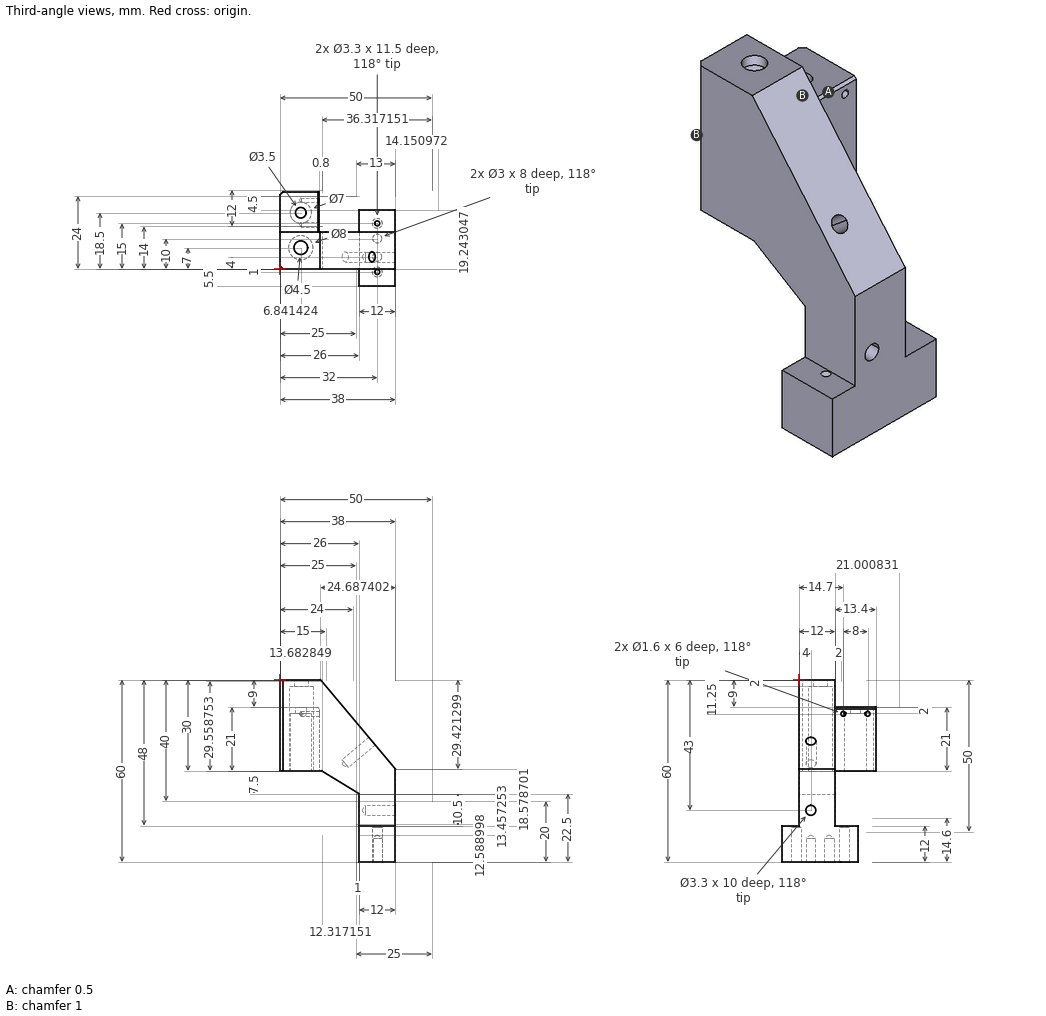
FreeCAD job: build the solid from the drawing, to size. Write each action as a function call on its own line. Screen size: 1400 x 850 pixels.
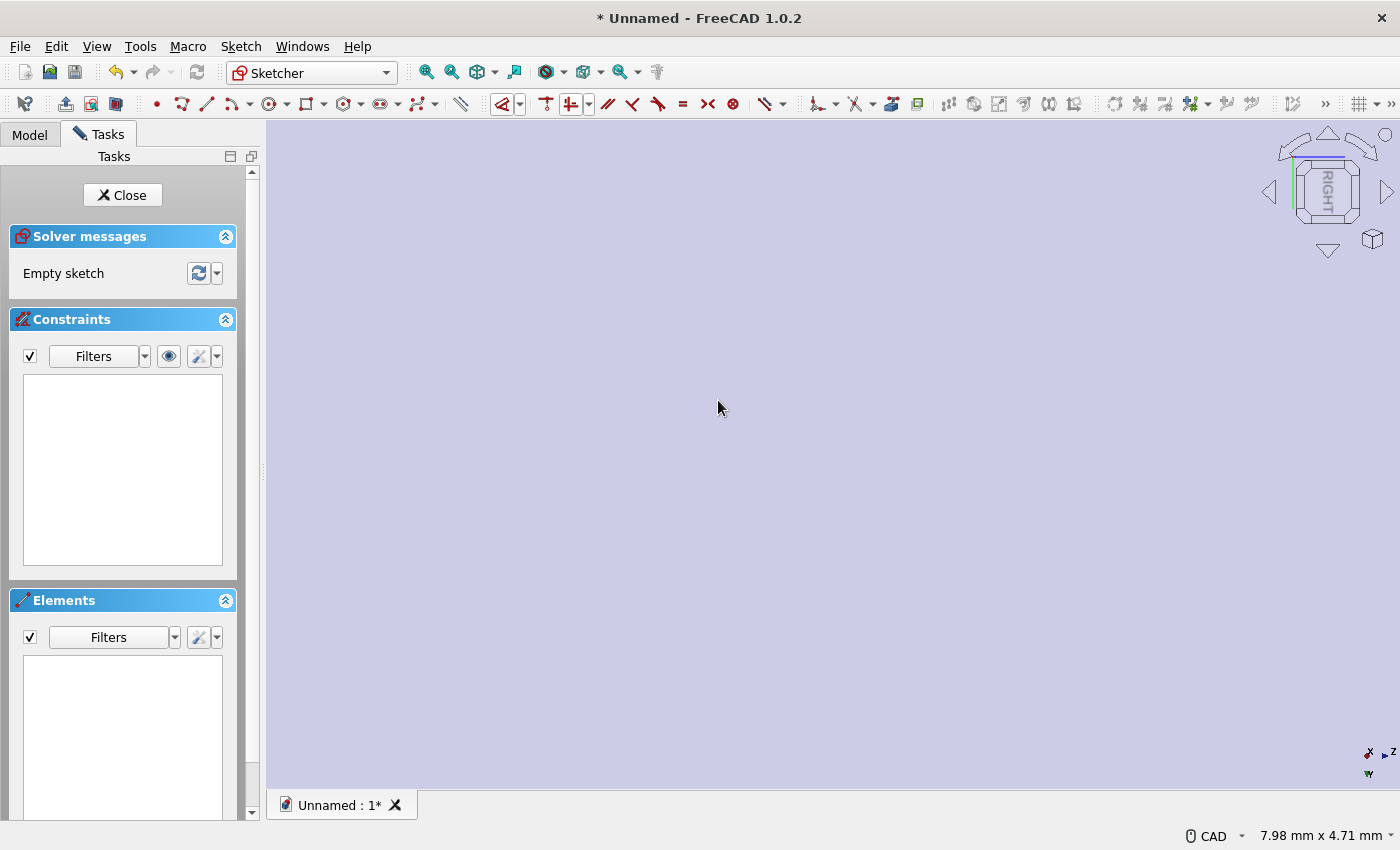
click(268, 104)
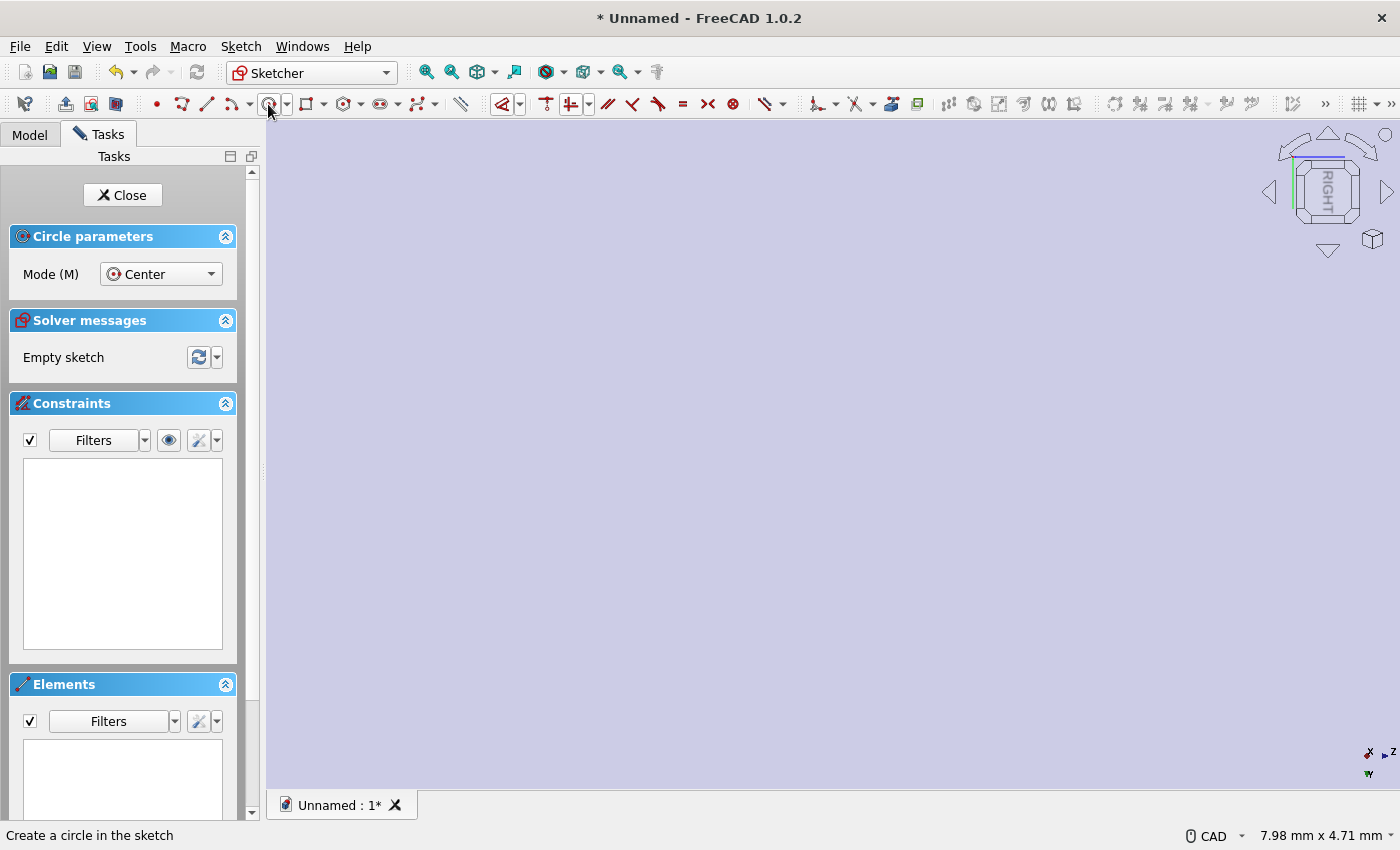
click(756, 445)
click(922, 279)
key(Escape)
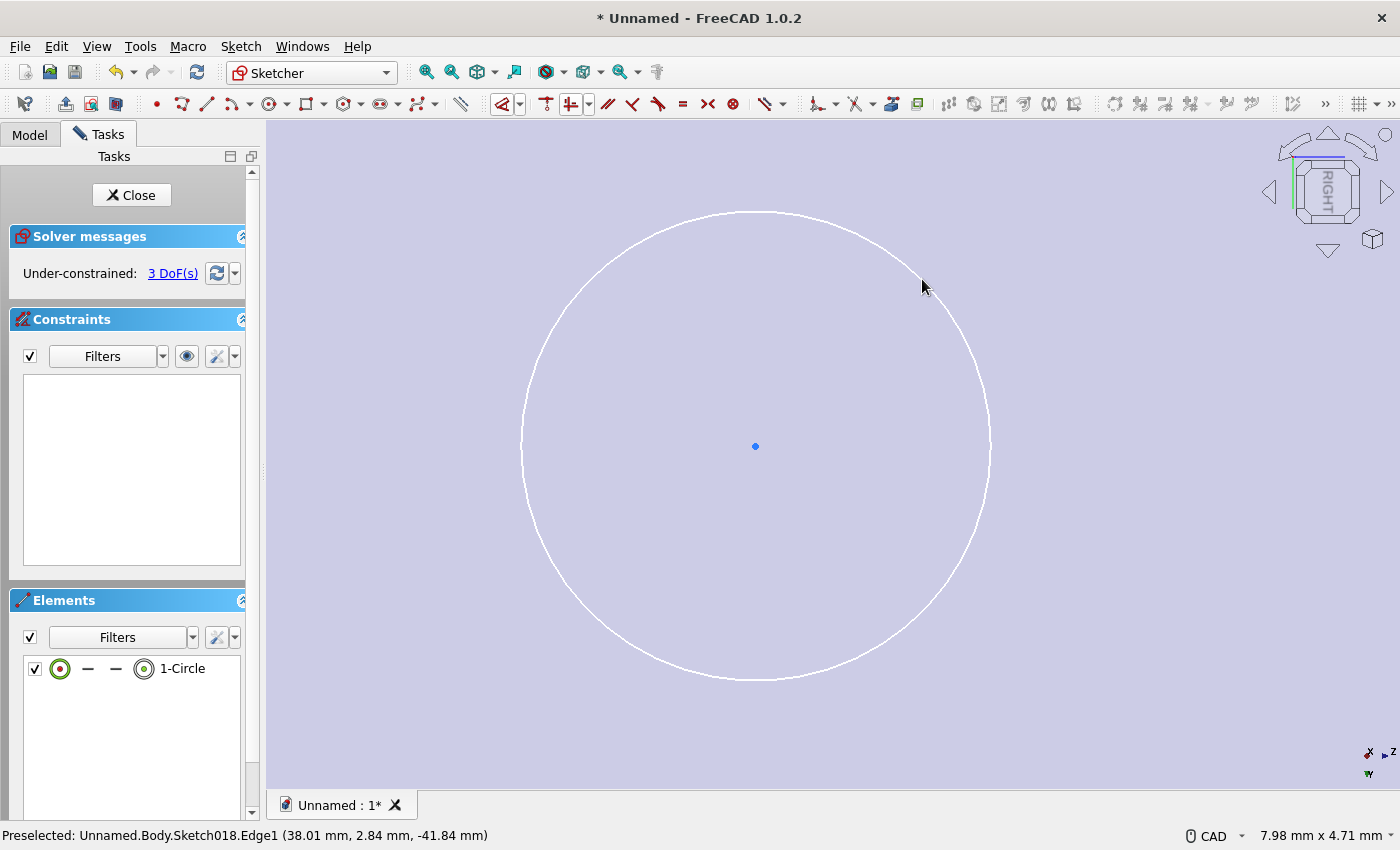
click(921, 279)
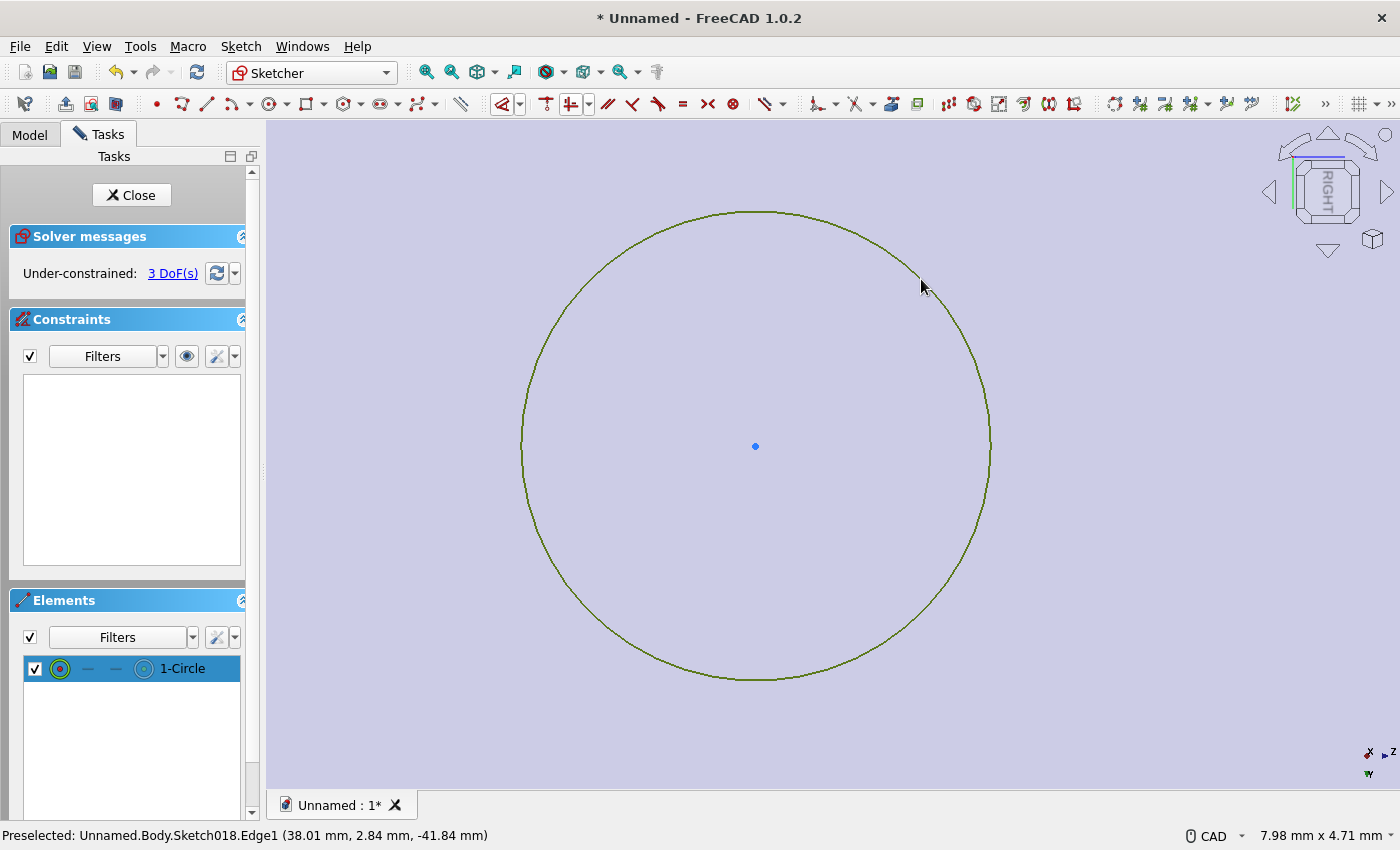
click(520, 104)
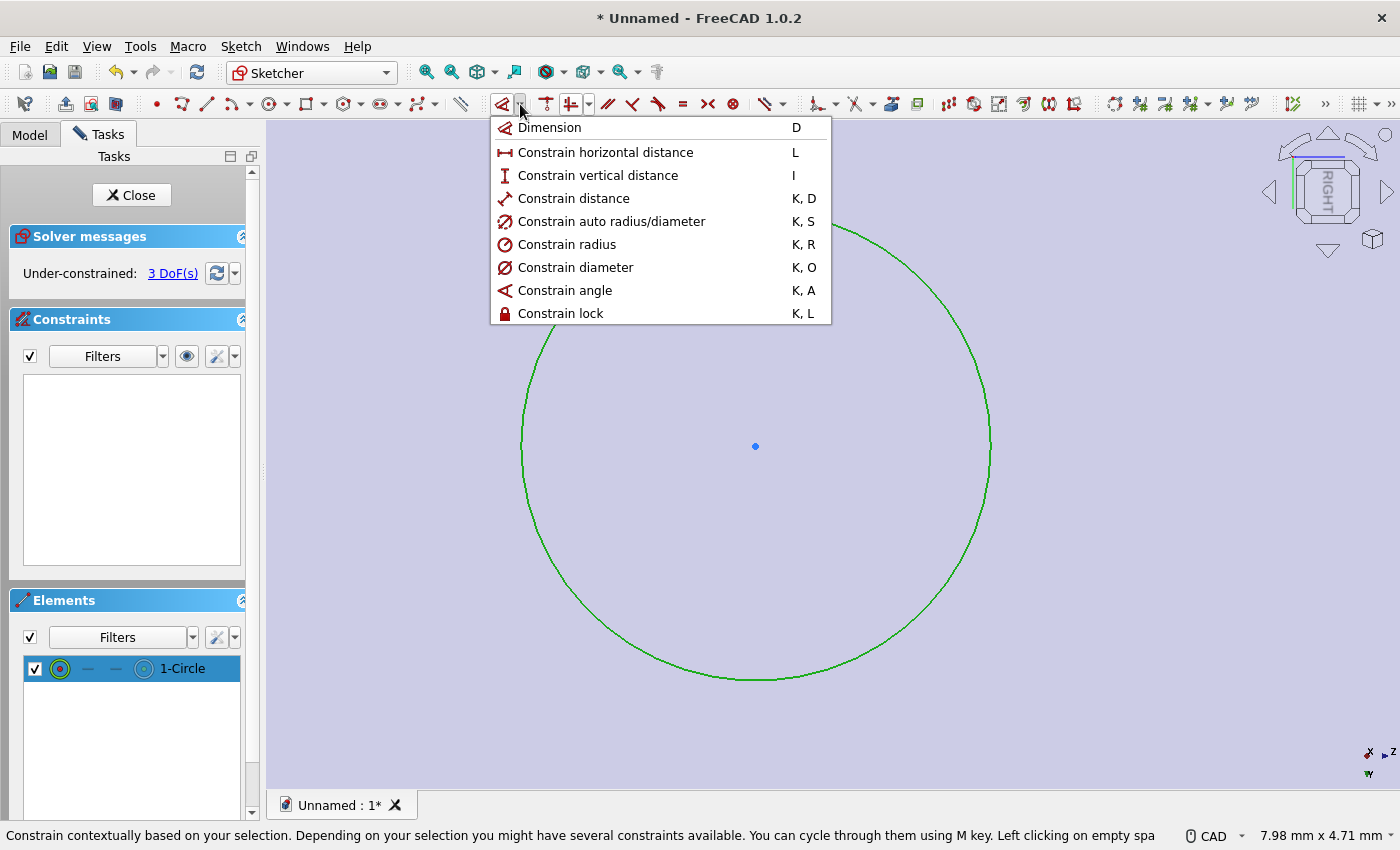
click(661, 268)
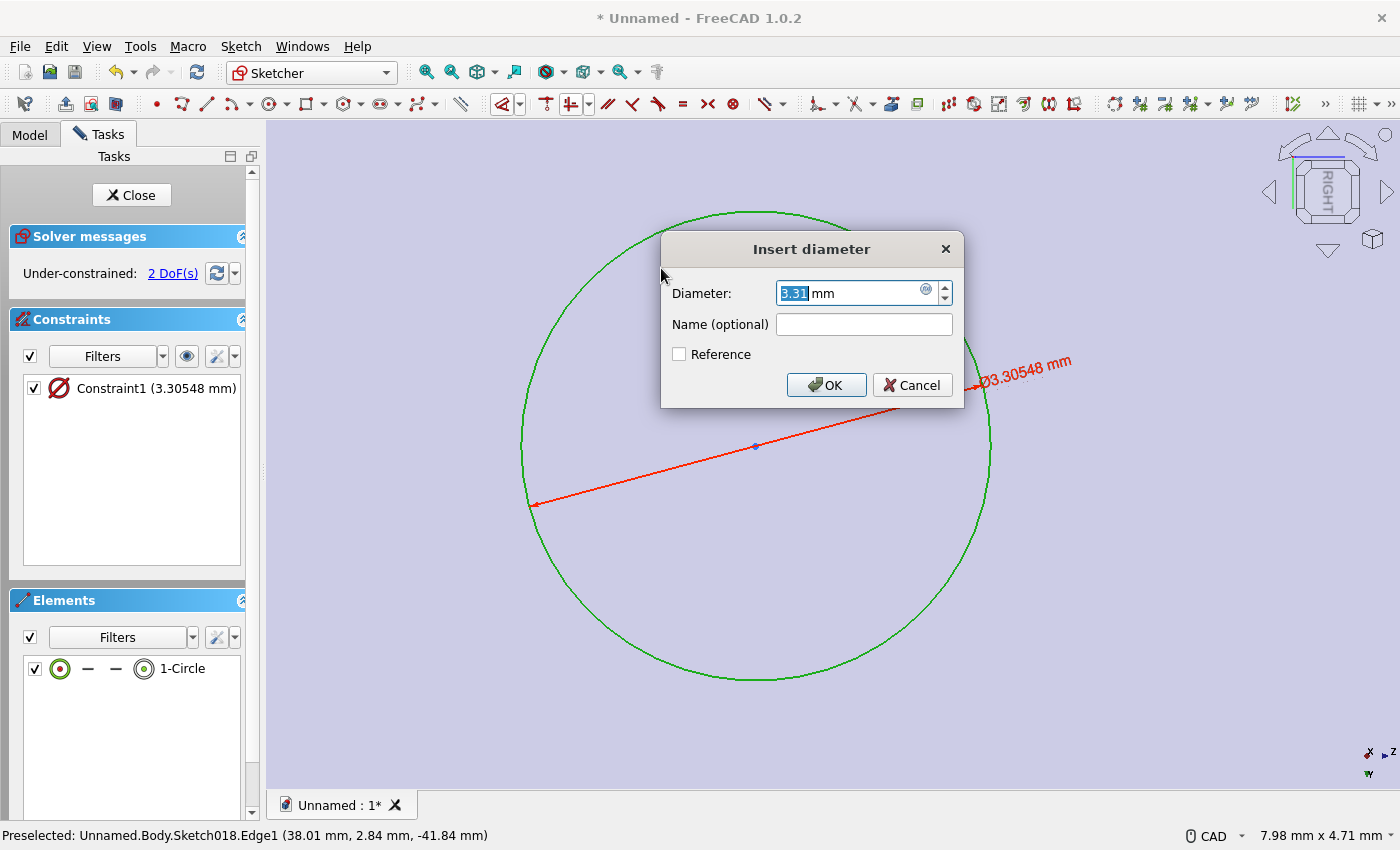
text(3.3)
key(Return)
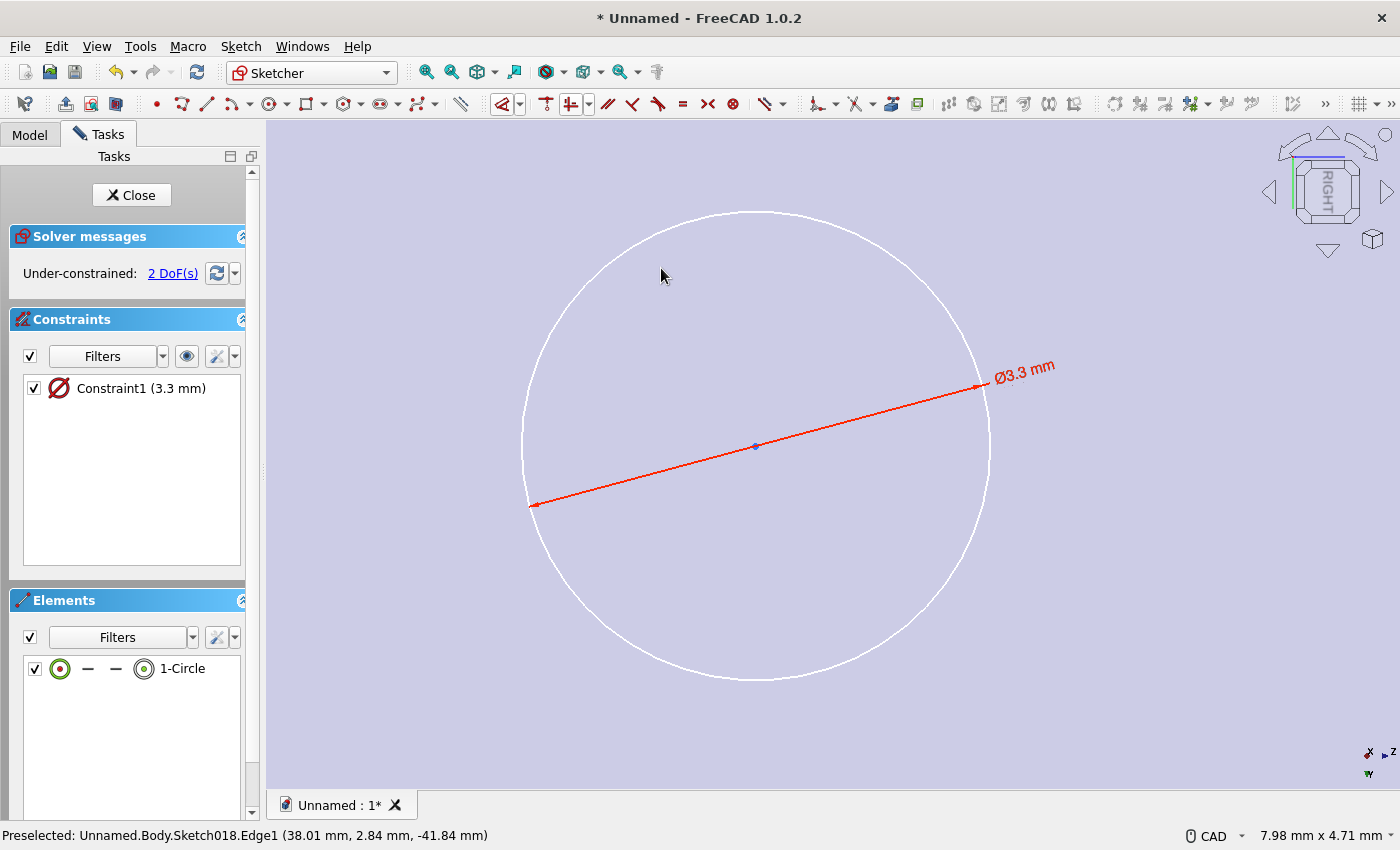
click(756, 446)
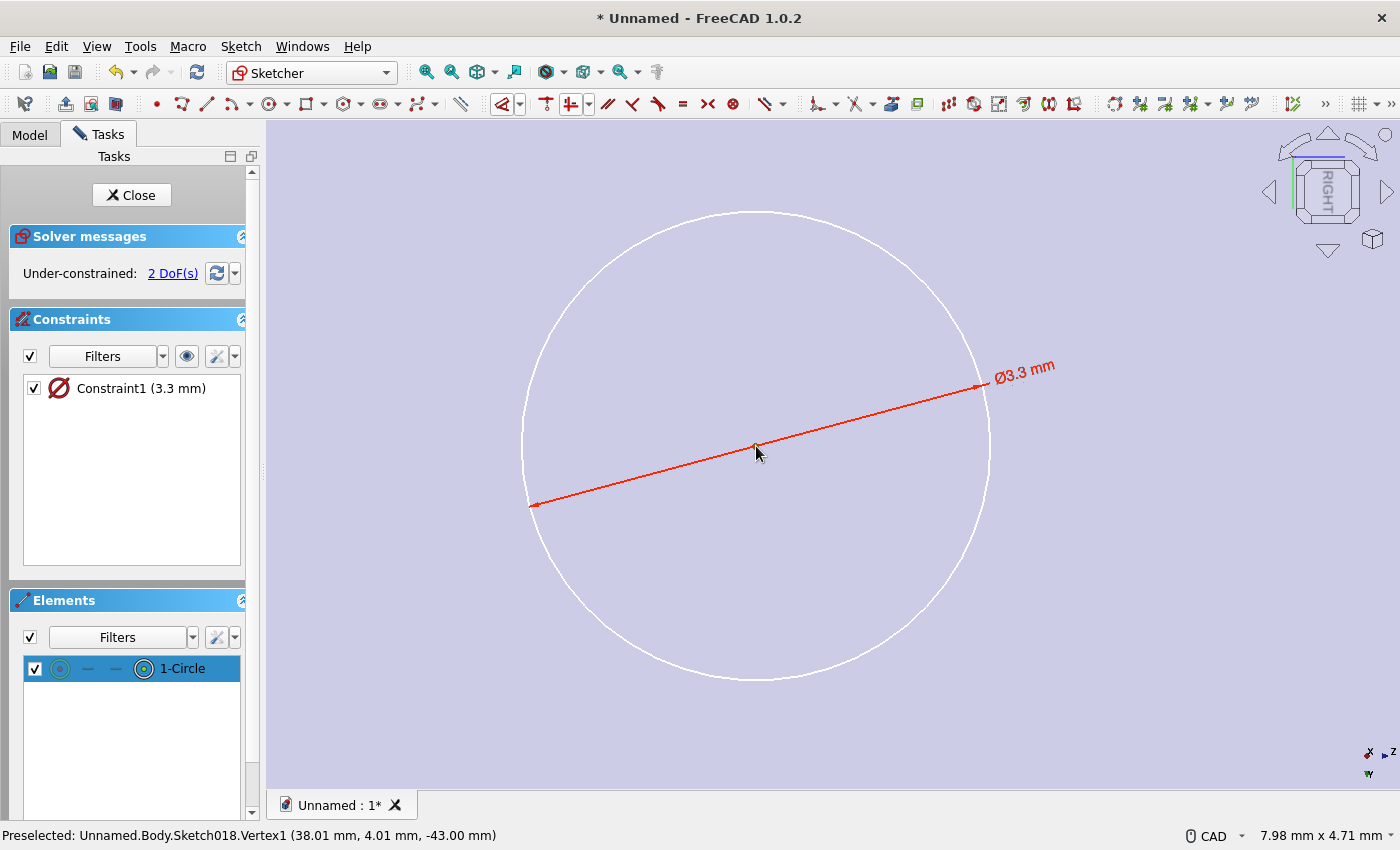
key(i)